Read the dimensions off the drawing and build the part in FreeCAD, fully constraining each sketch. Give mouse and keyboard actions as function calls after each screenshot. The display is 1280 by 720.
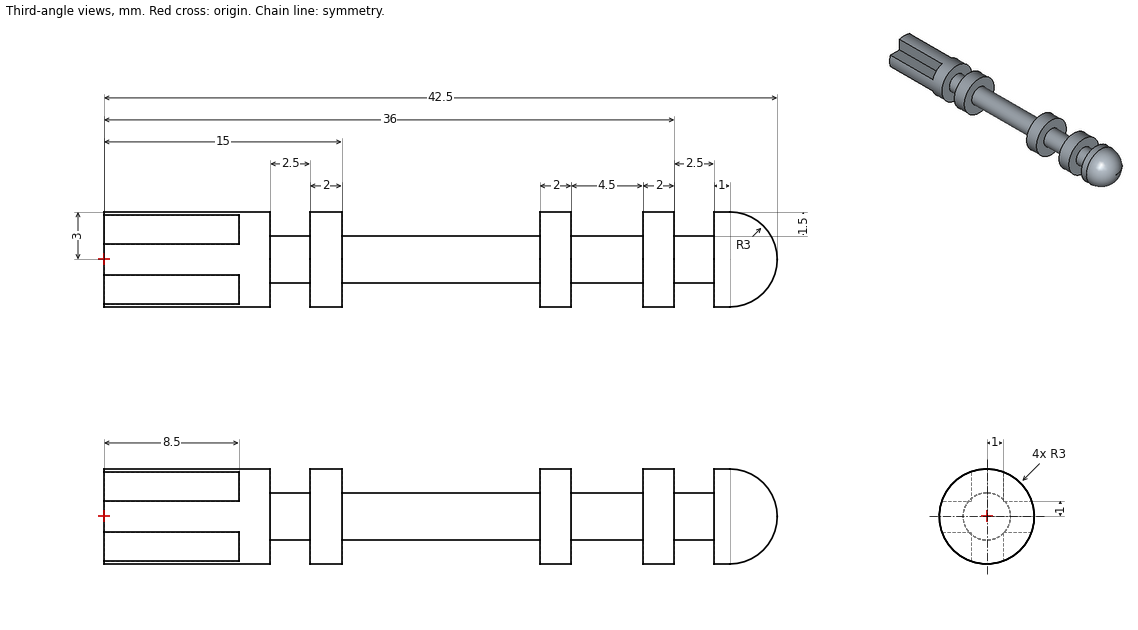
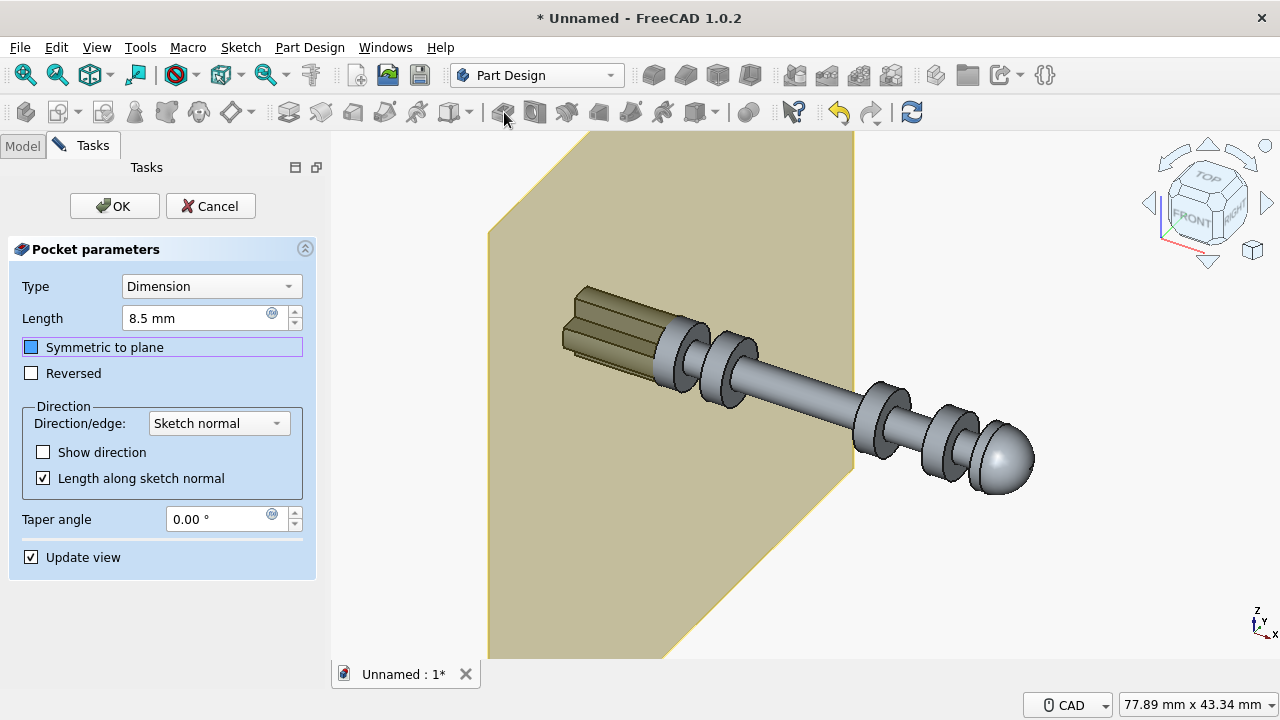
click(115, 206)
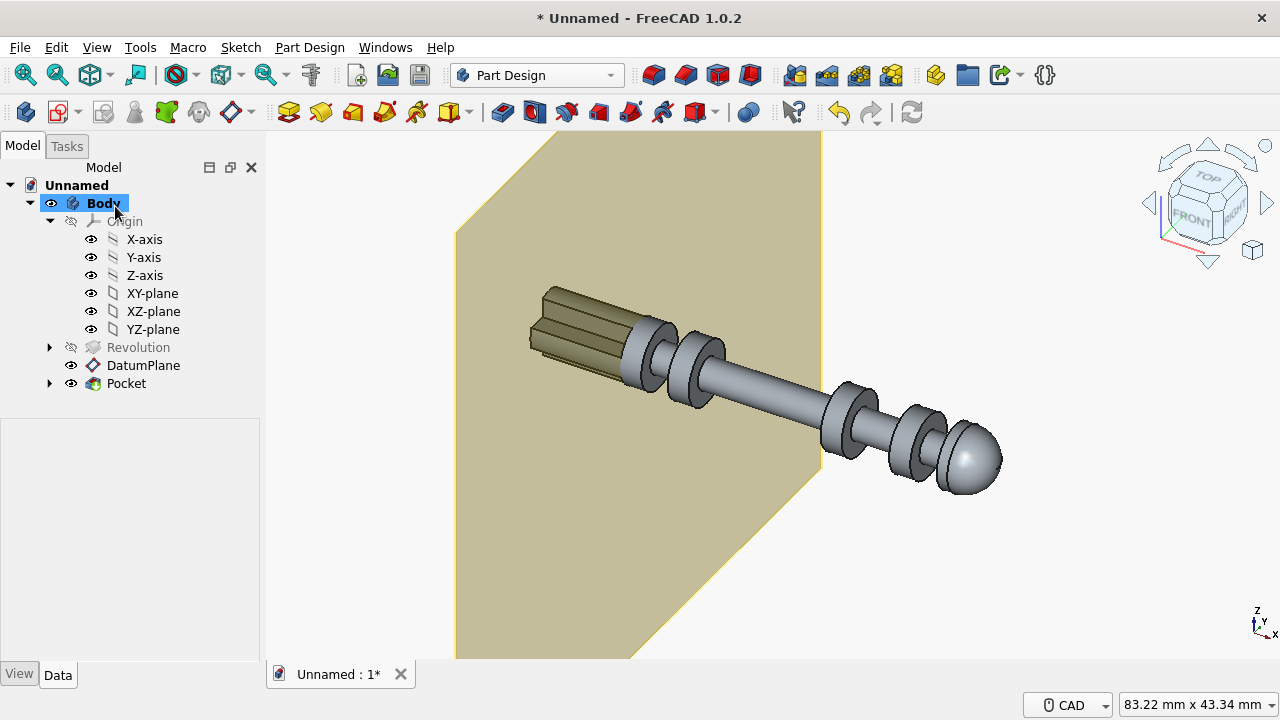
click(116, 365)
key(space)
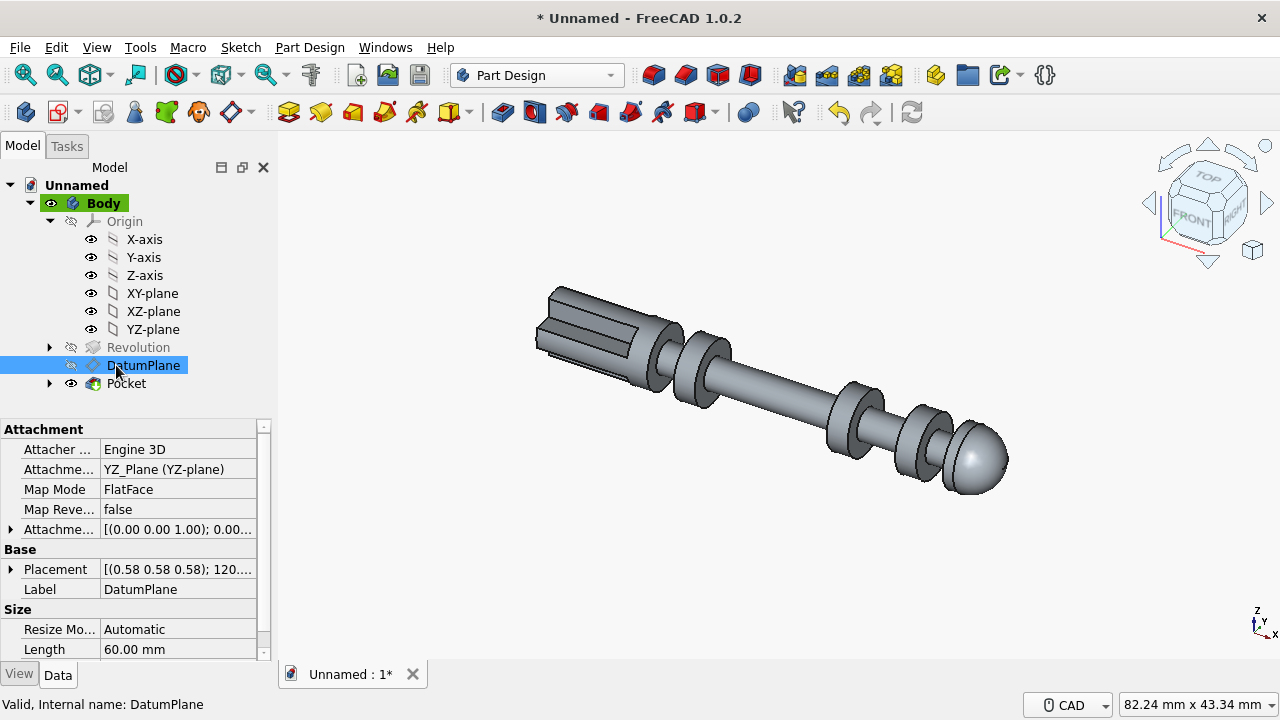
key(0)